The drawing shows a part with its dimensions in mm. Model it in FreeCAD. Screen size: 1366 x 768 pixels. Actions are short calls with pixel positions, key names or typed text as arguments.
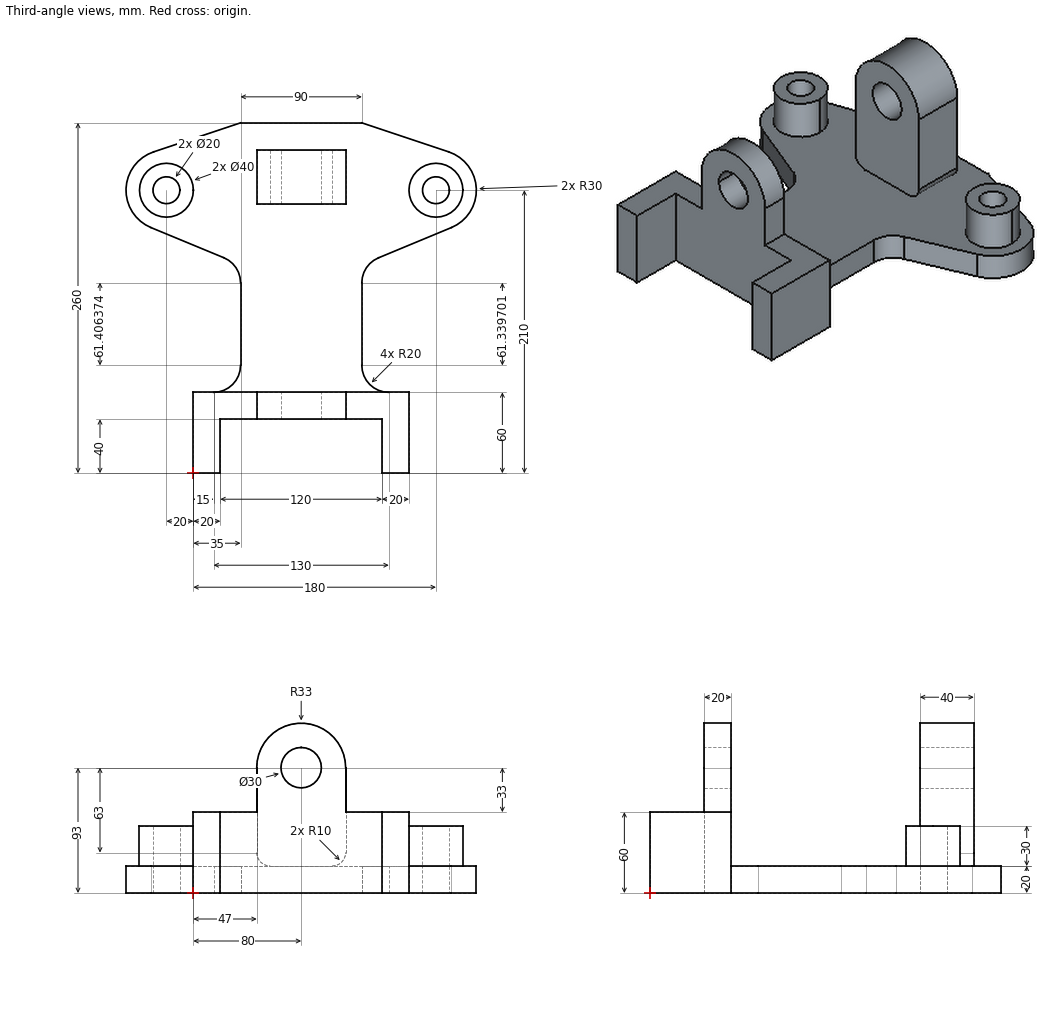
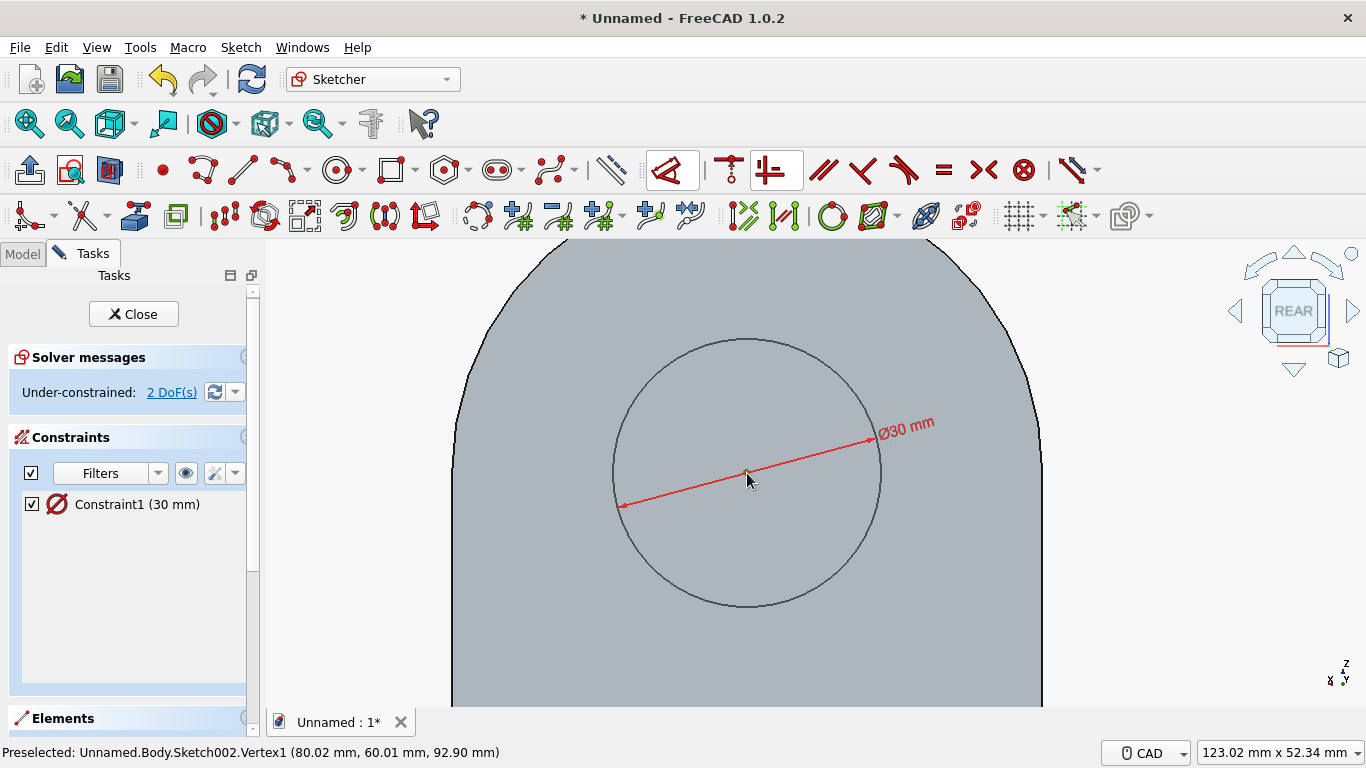
click(694, 170)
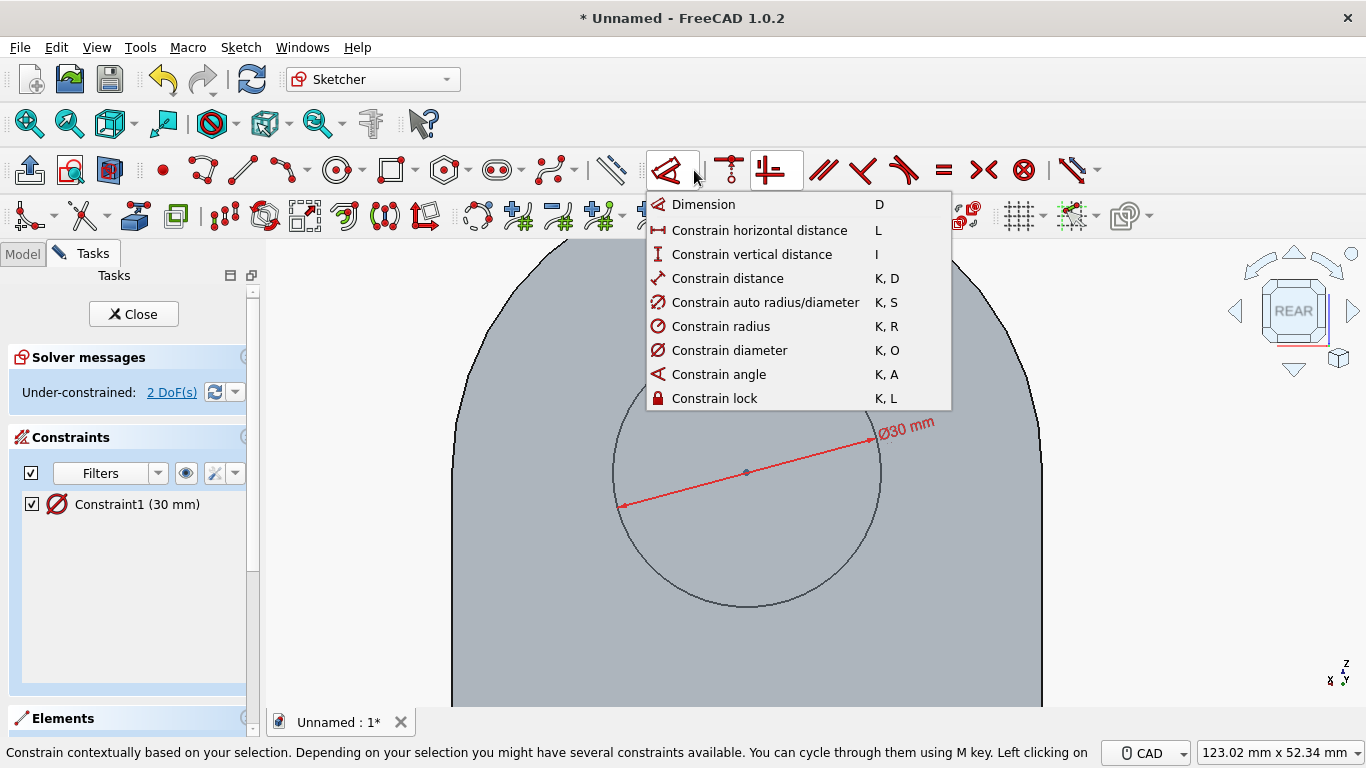
click(799, 230)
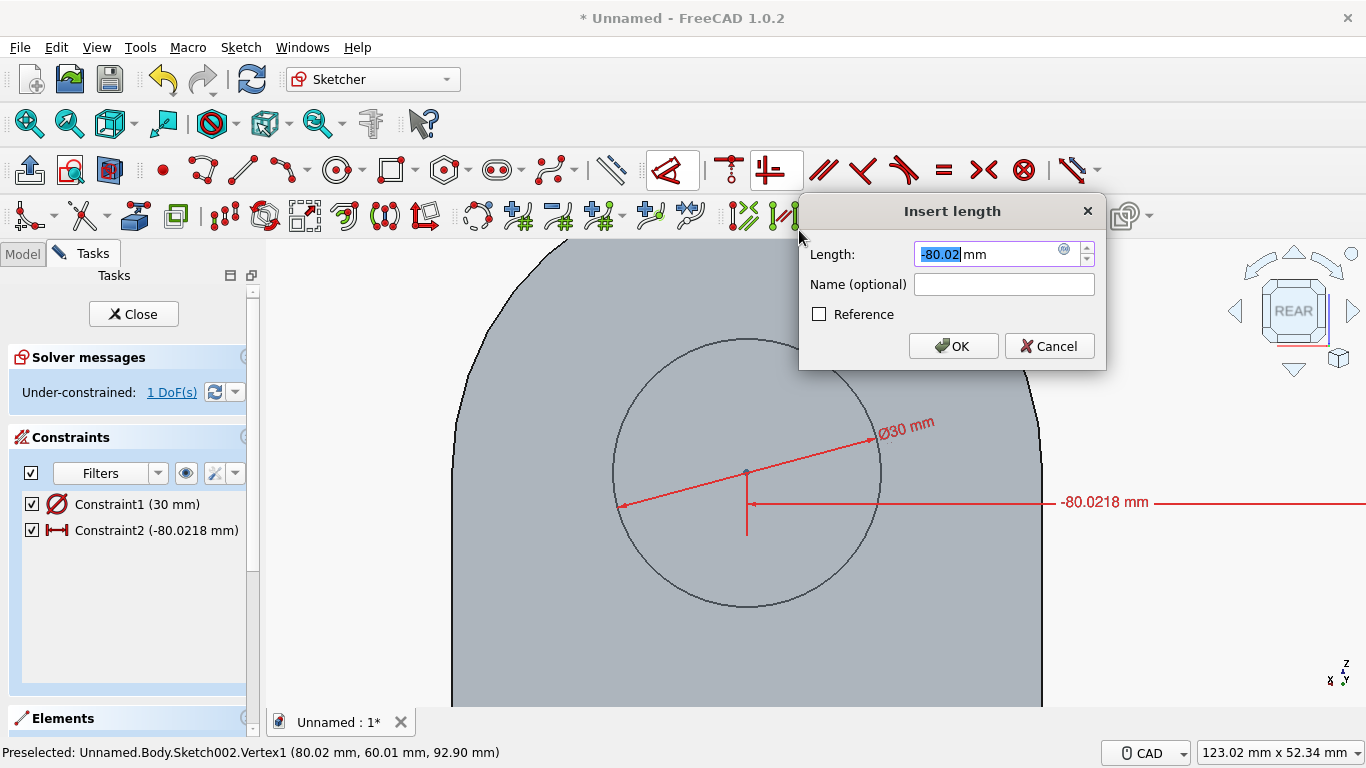
text(-80)
key(Return)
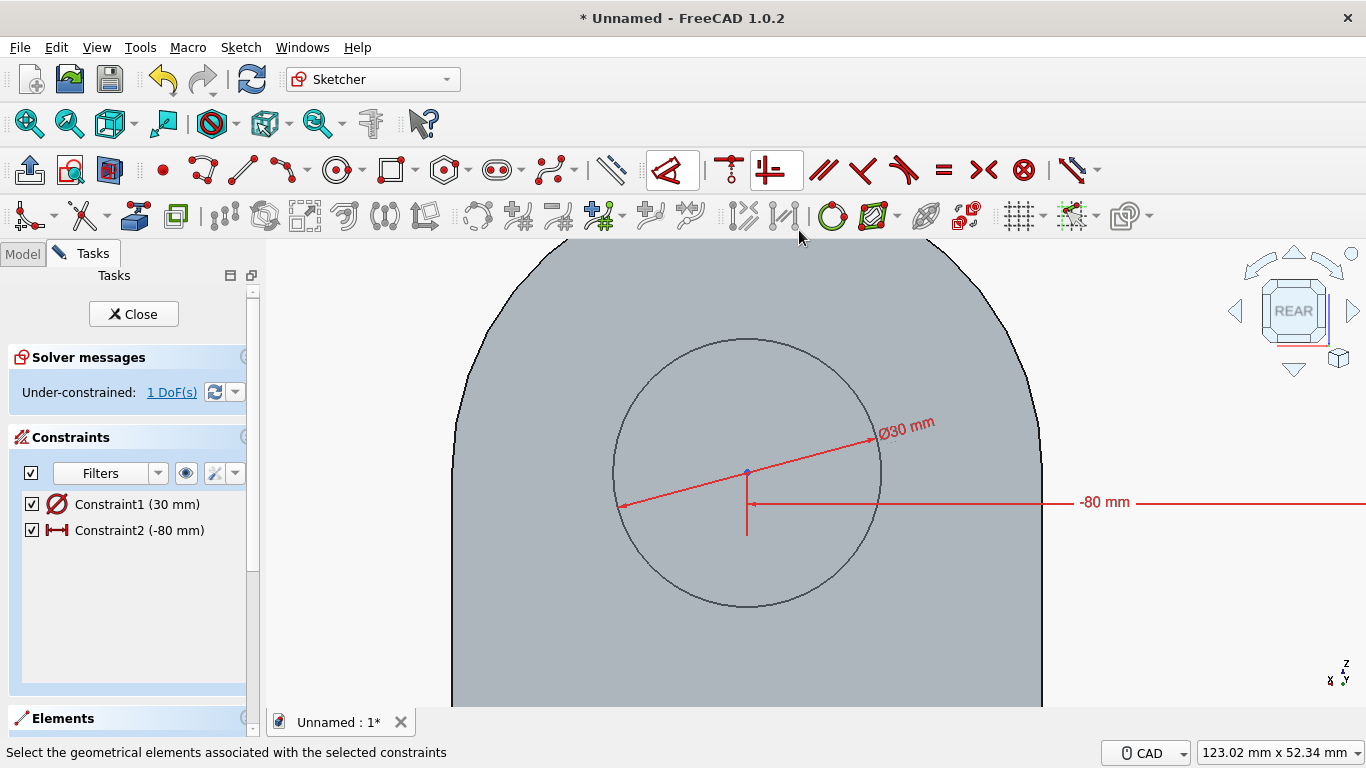
click(747, 473)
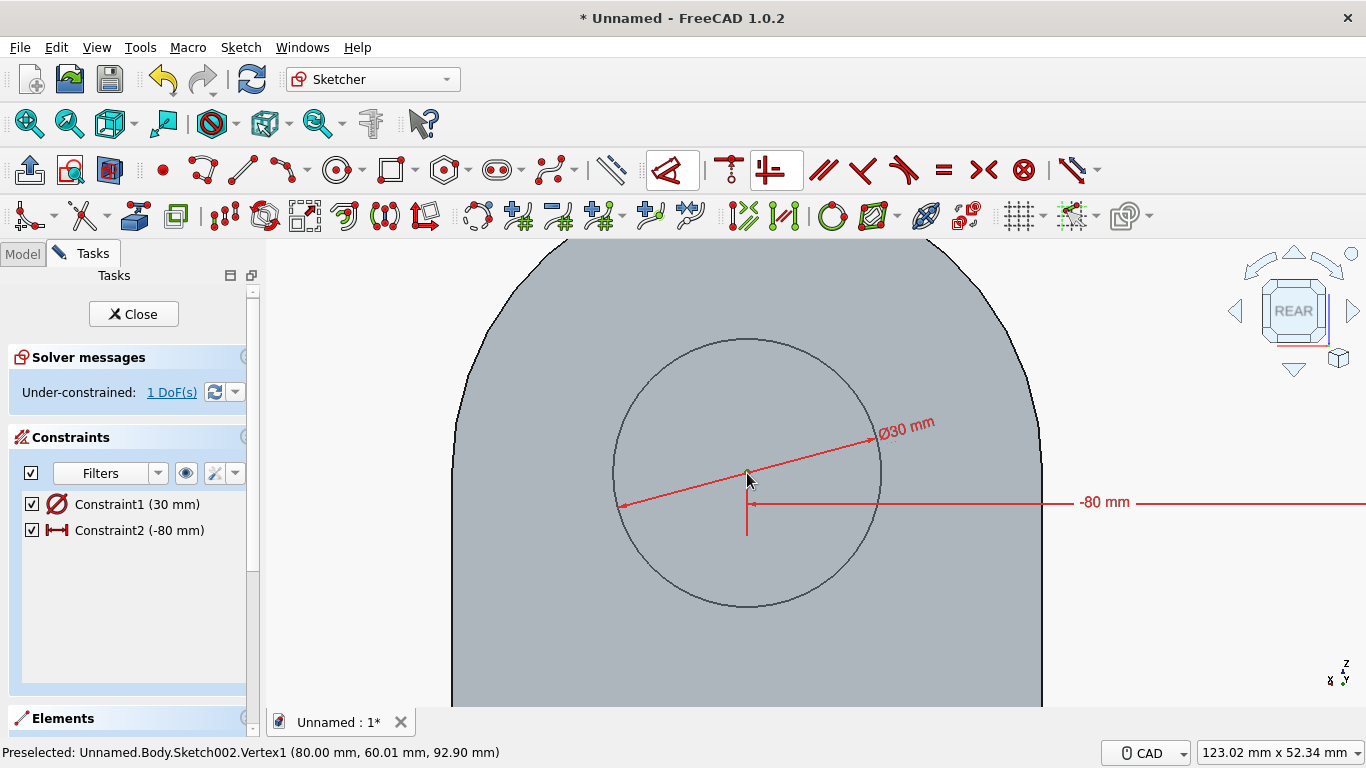
click(694, 170)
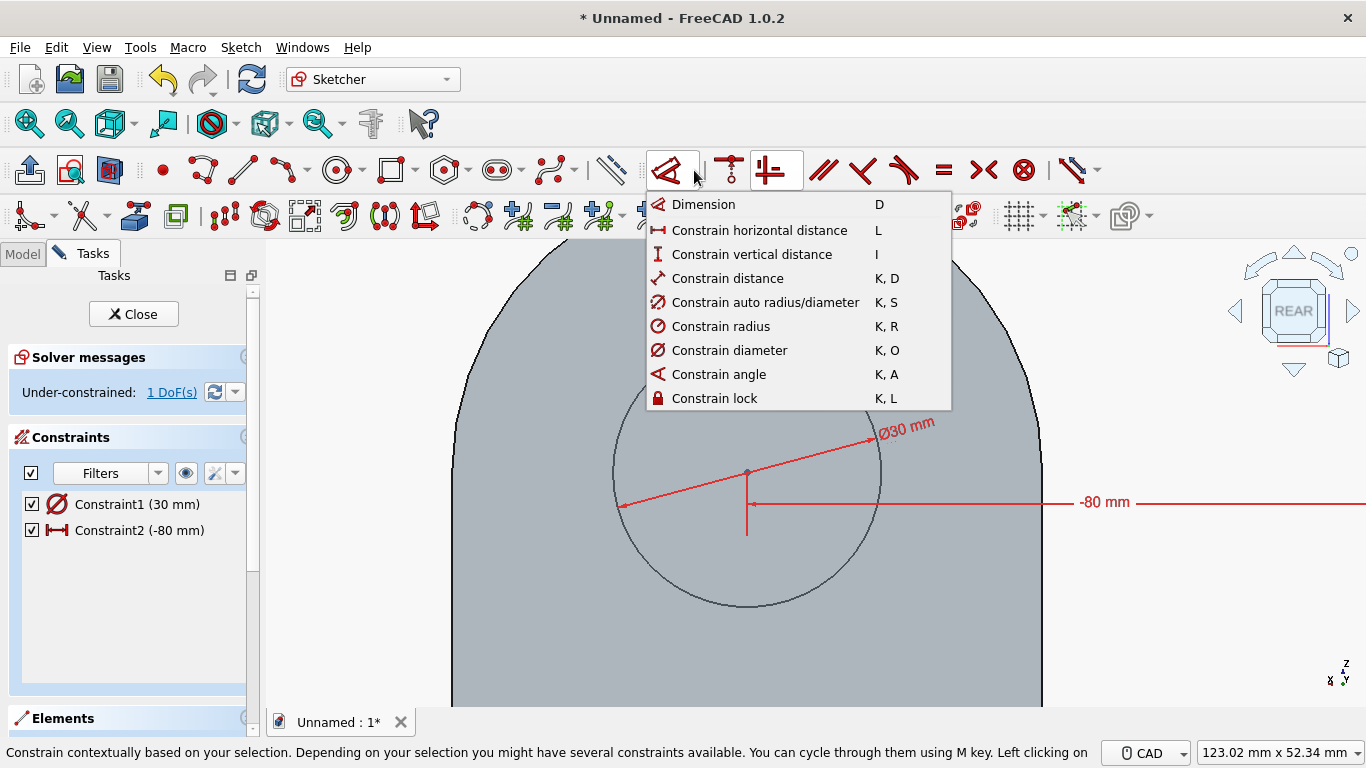
click(799, 254)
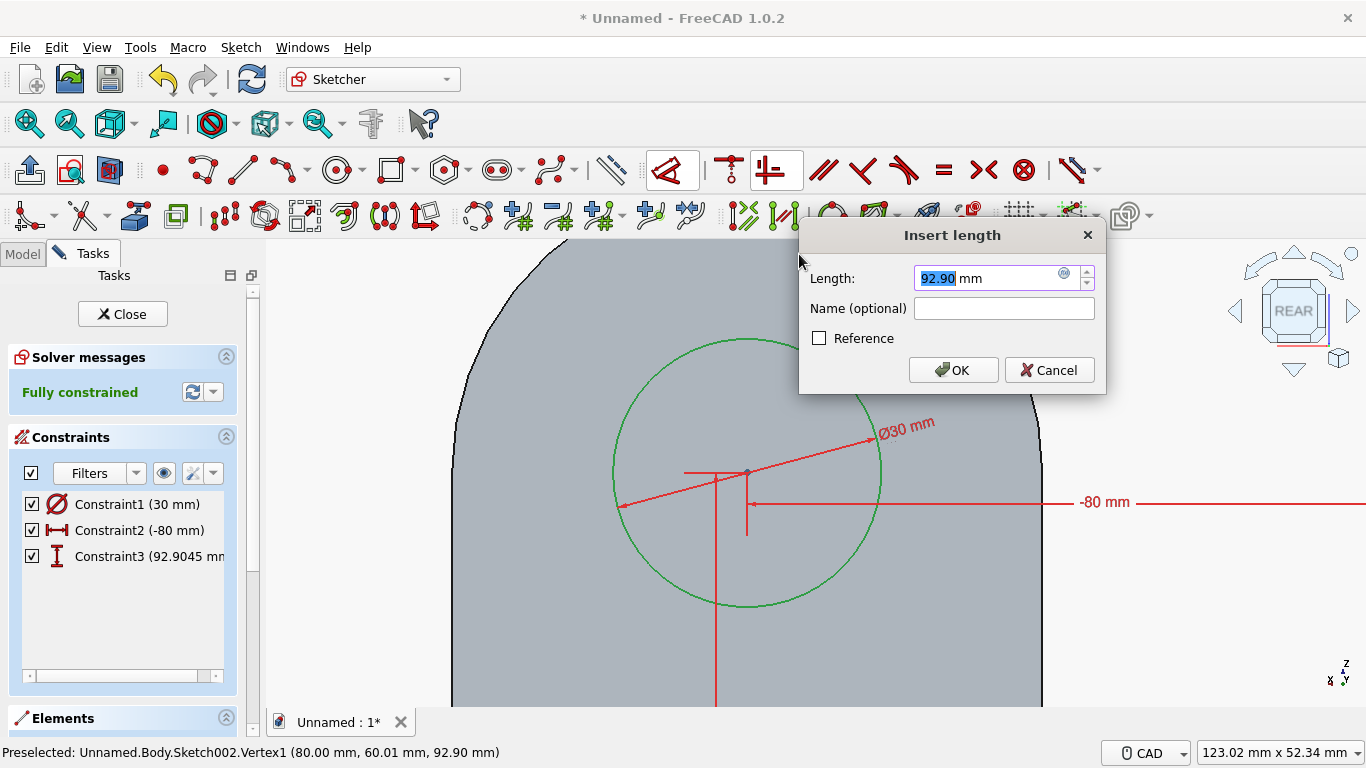
text(93)
key(Return)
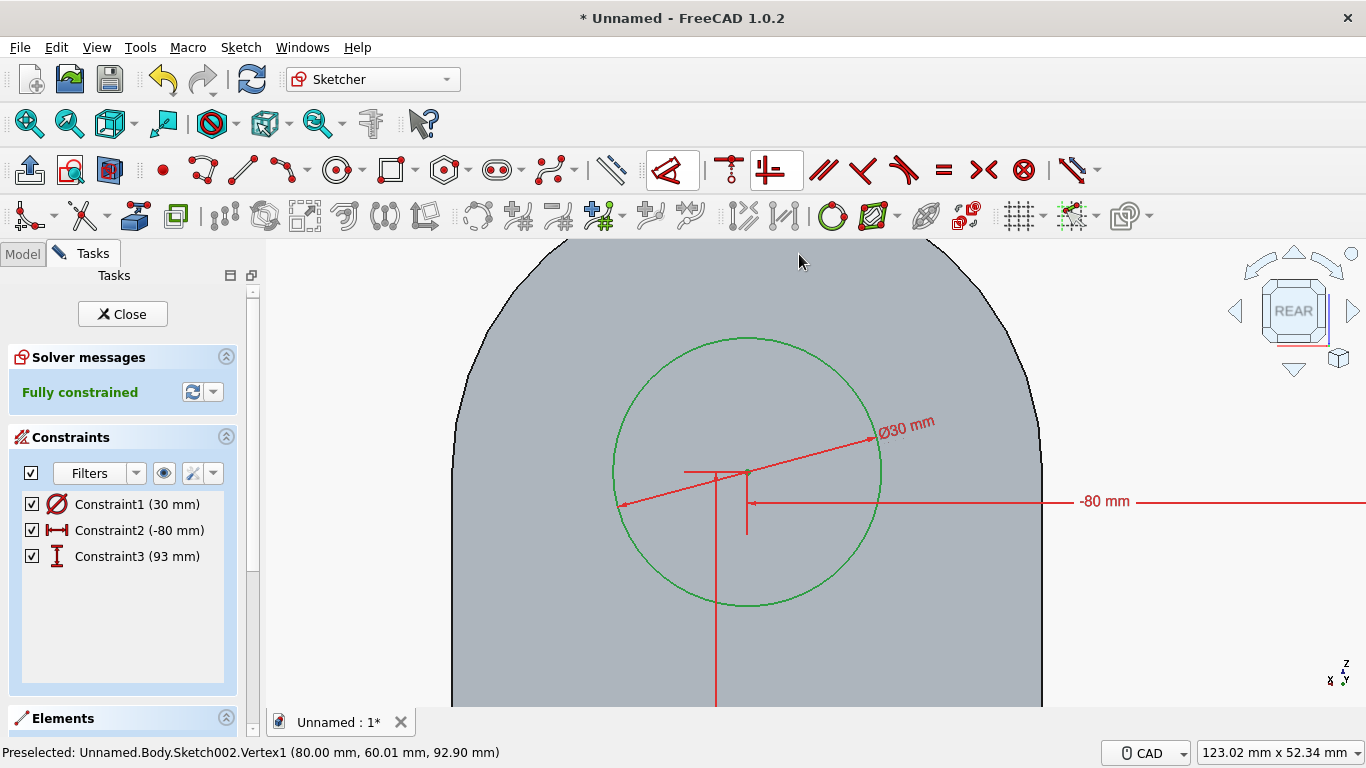
click(123, 314)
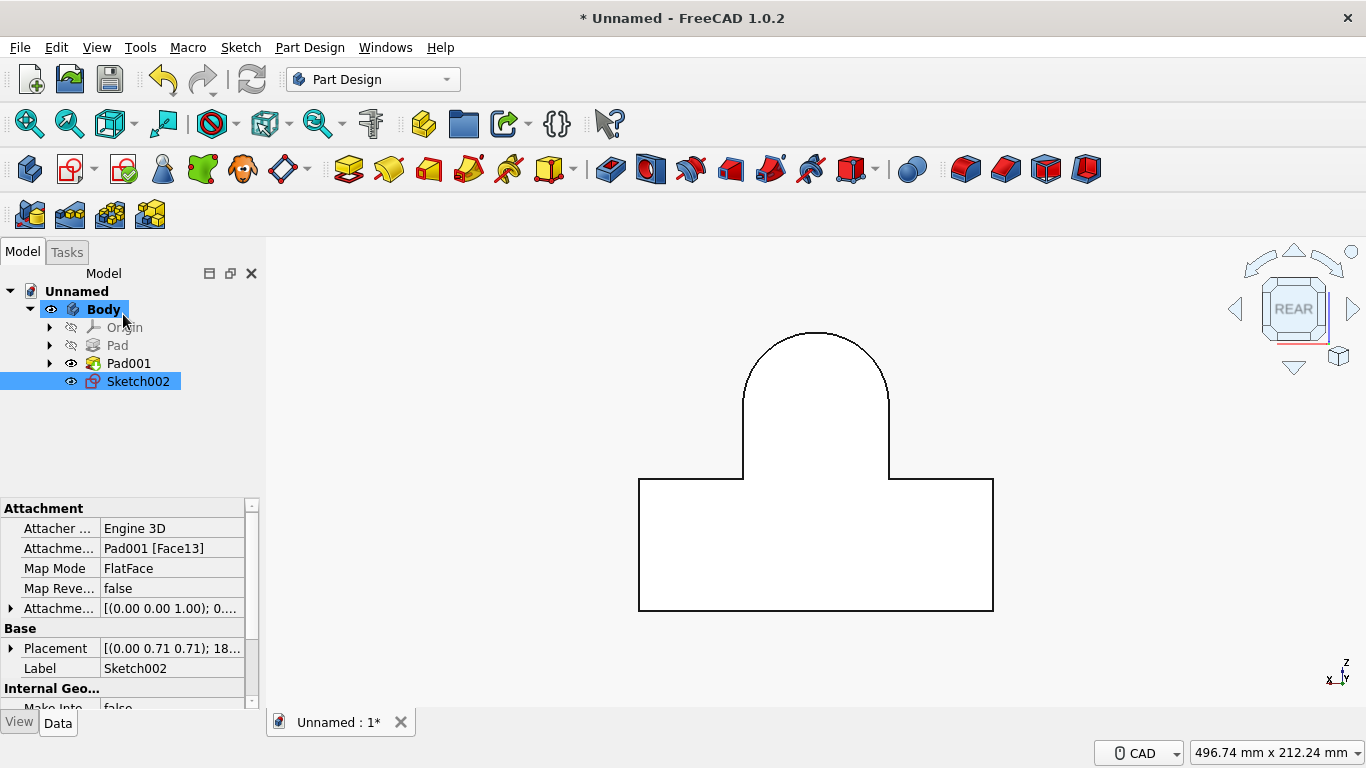
click(612, 170)